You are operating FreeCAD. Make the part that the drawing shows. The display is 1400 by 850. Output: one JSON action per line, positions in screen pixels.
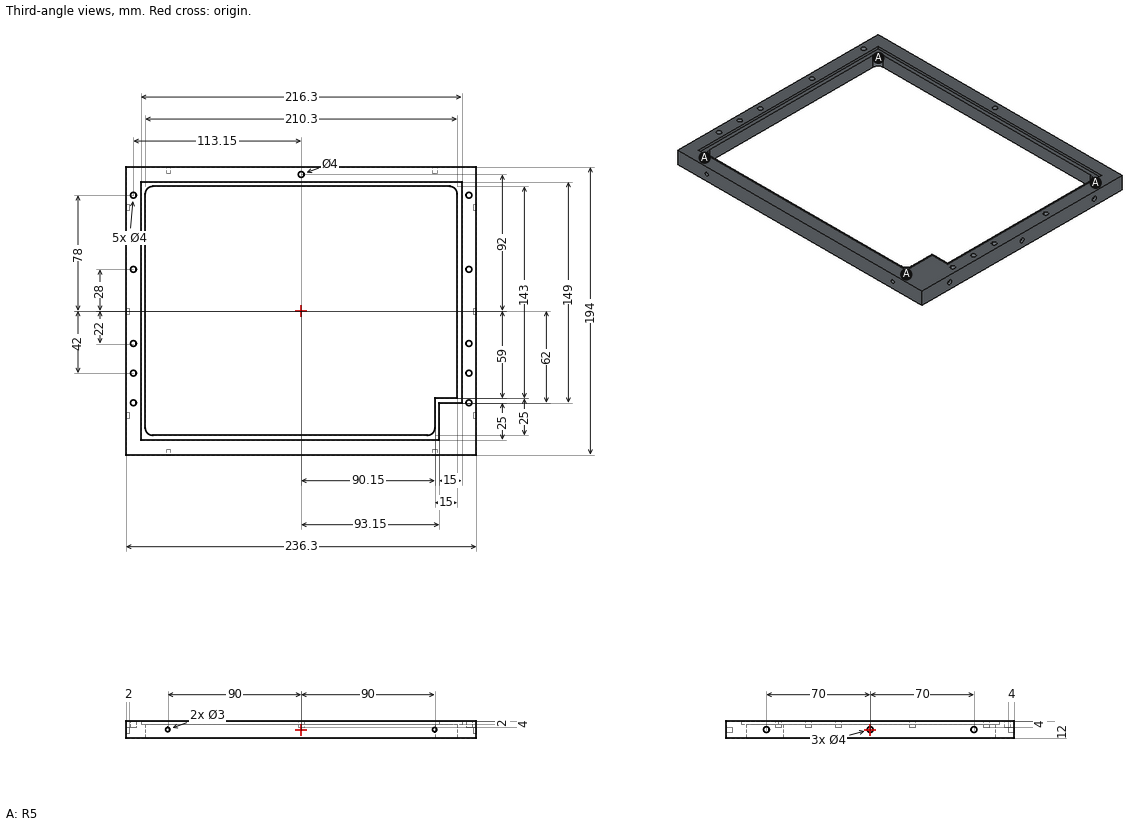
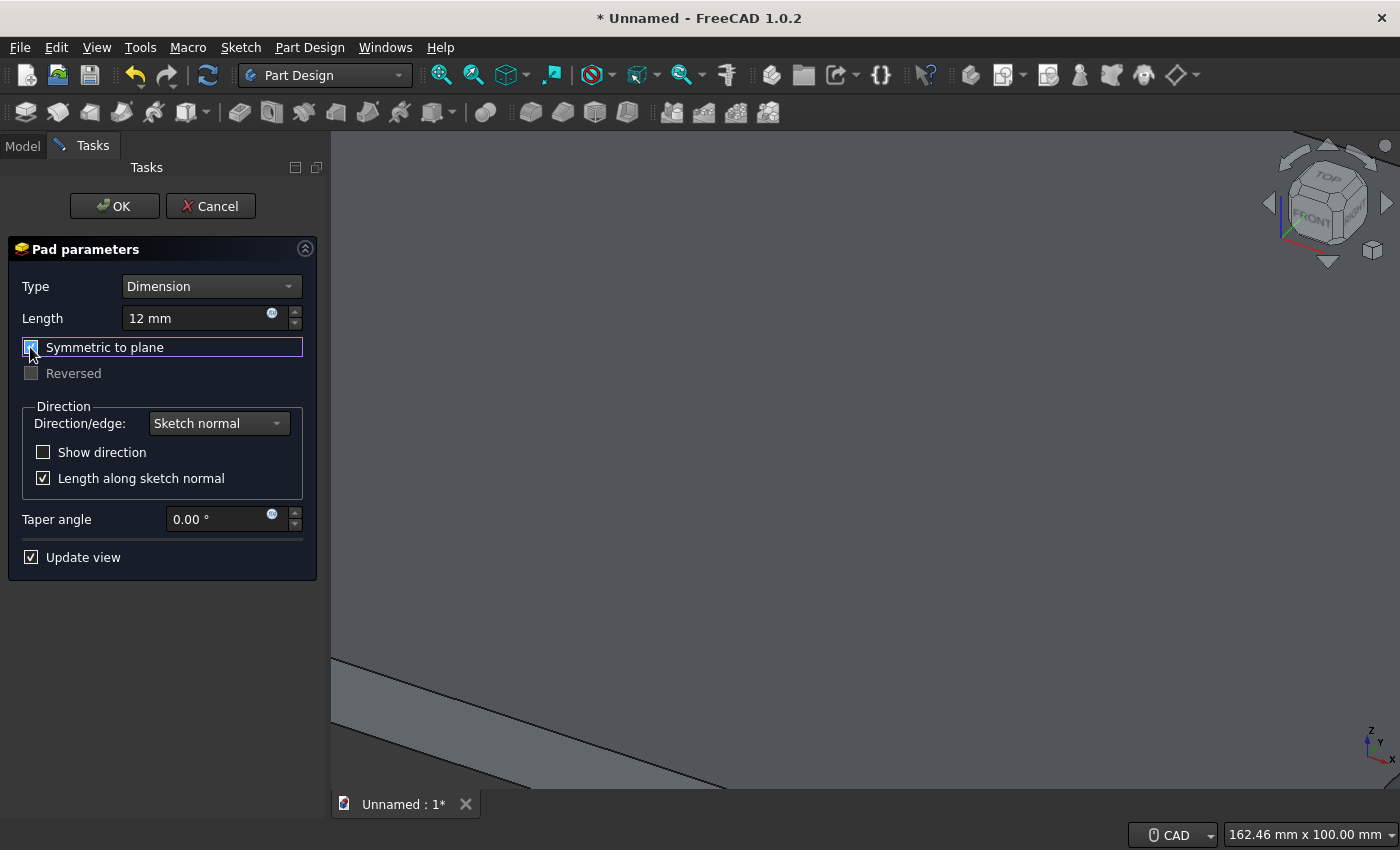
{"action": "left_click", "coordinate": [115, 206]}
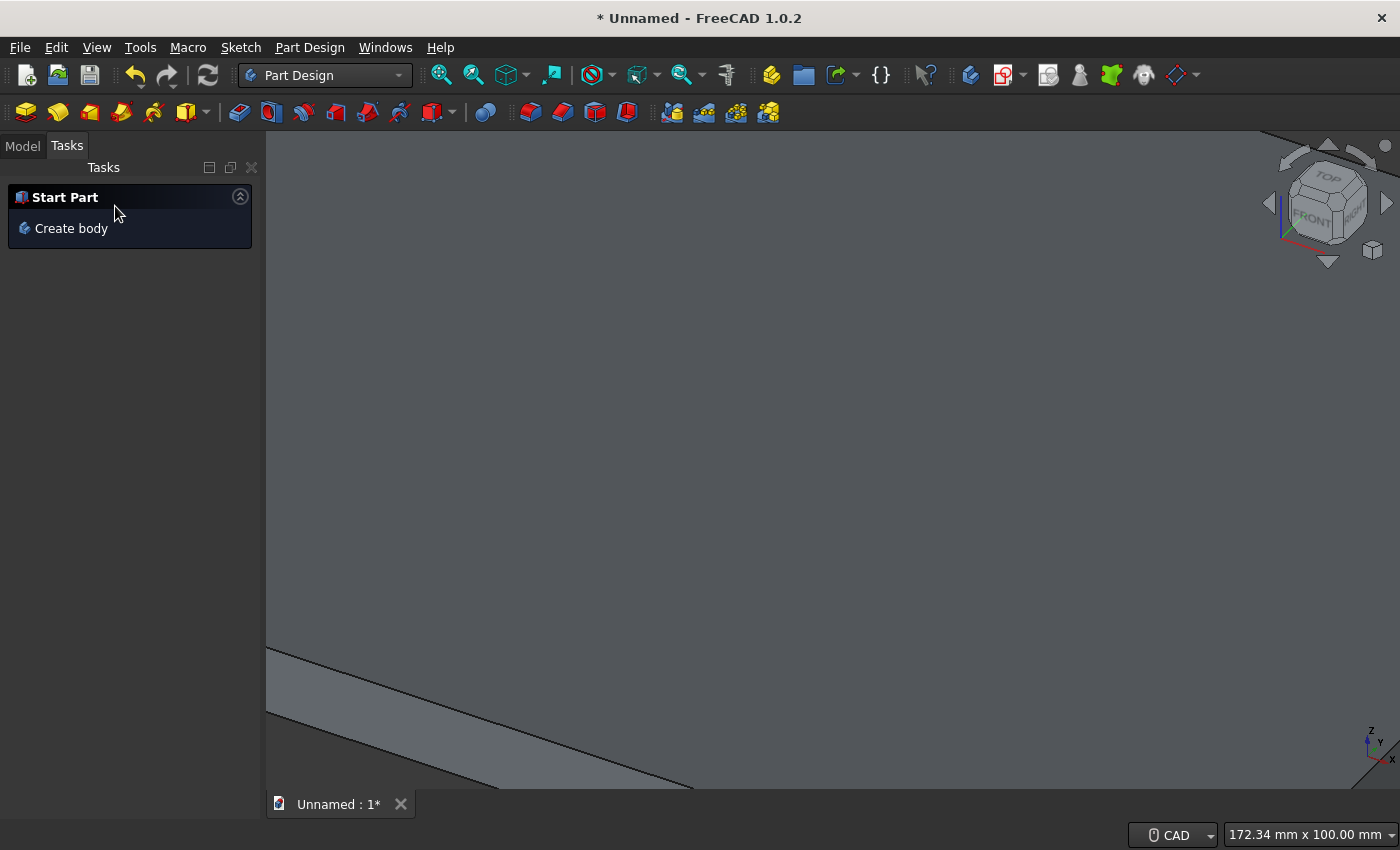
{"action": "left_click", "coordinate": [442, 76]}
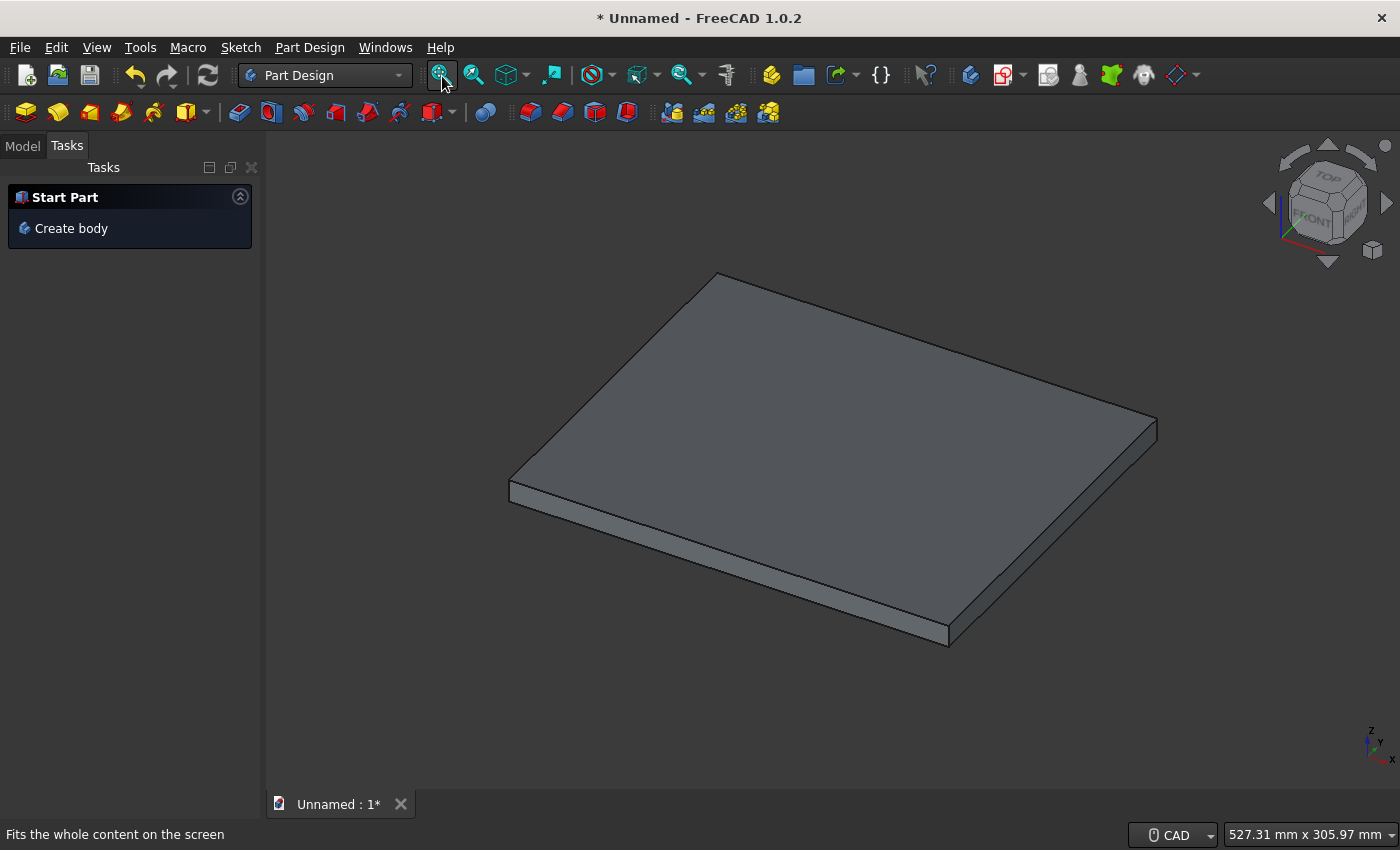
{"action": "left_click", "coordinate": [833, 448]}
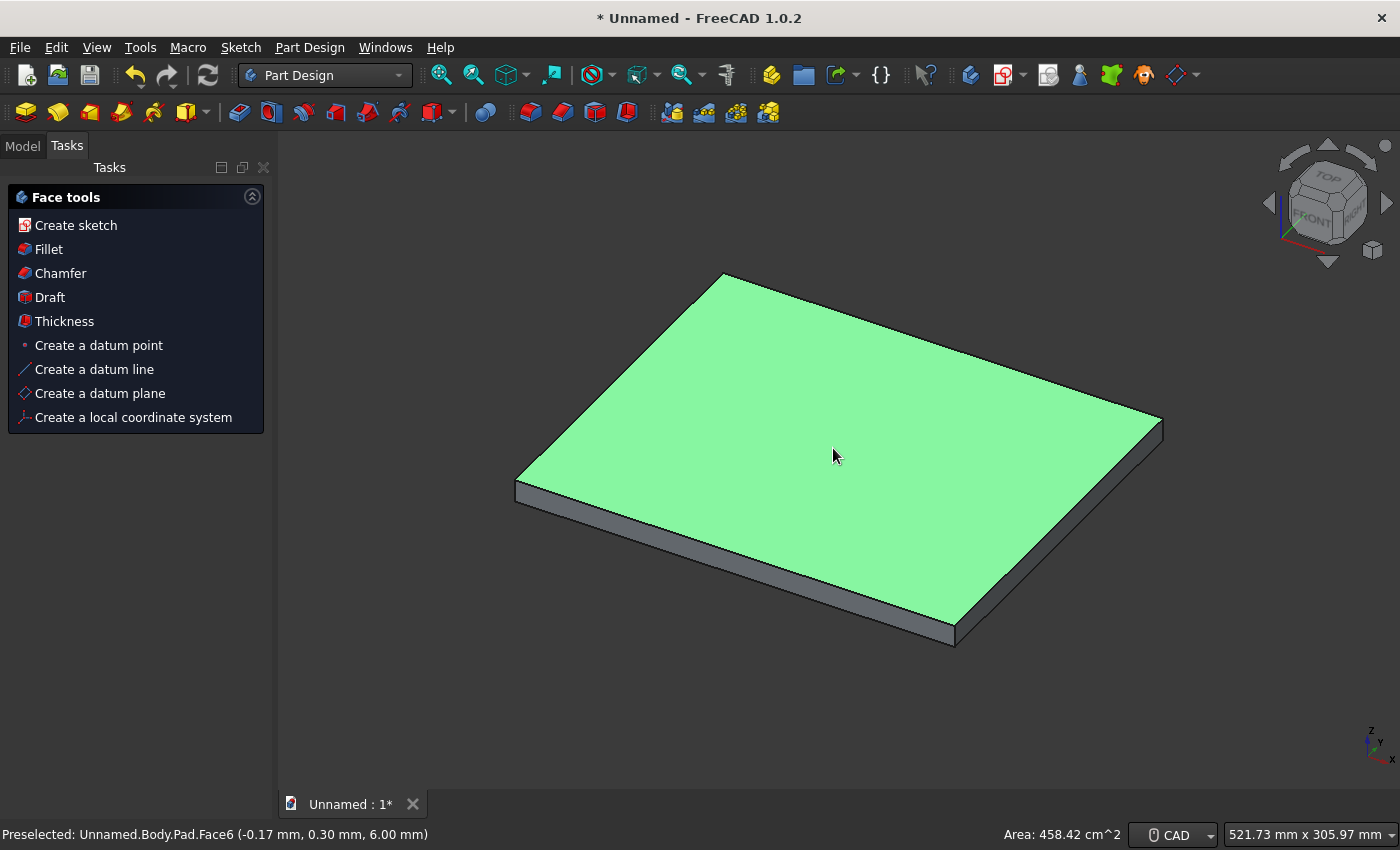
{"action": "left_click", "coordinate": [1004, 76]}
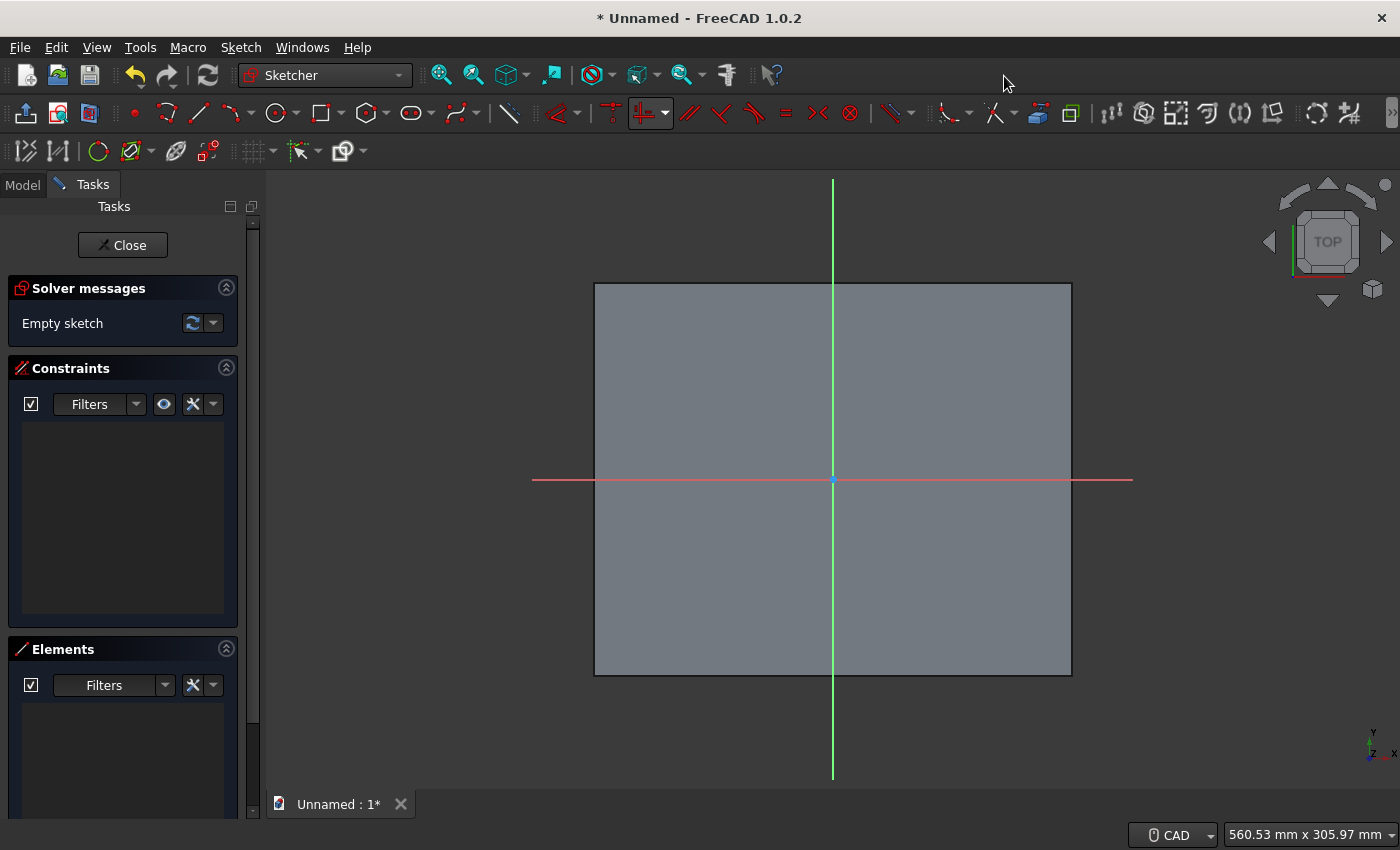
{"action": "left_click", "coordinate": [168, 114]}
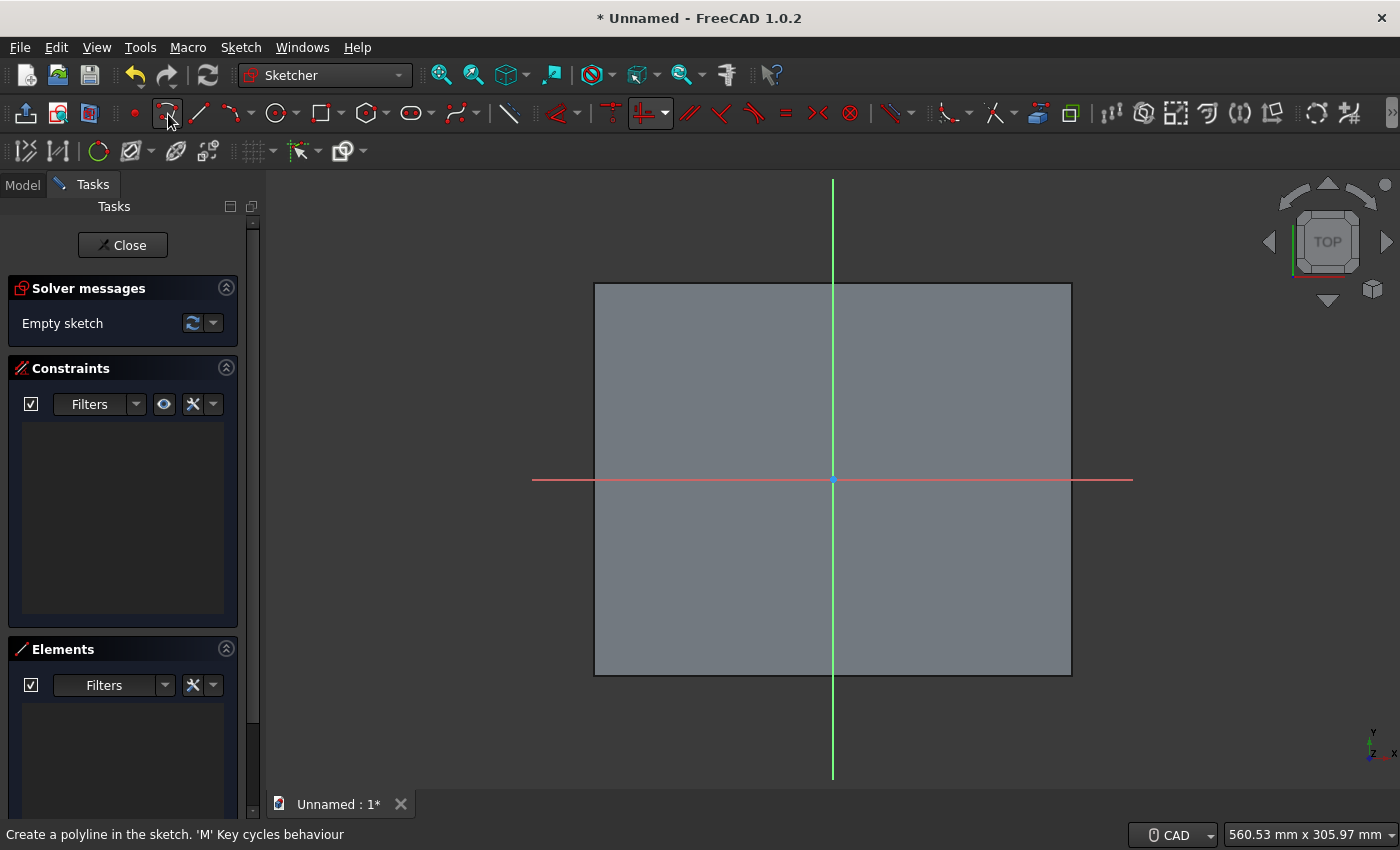
{"action": "left_click", "coordinate": [1021, 605]}
{"action": "left_click", "coordinate": [1052, 605]}
{"action": "left_click", "coordinate": [1052, 303]}
{"action": "left_click", "coordinate": [614, 303]}
{"action": "left_click", "coordinate": [614, 656]}
{"action": "left_click", "coordinate": [1021, 656]}
{"action": "left_click", "coordinate": [1021, 606]}
{"action": "key", "text": "Escape"}
{"action": "key", "text": "Escape"}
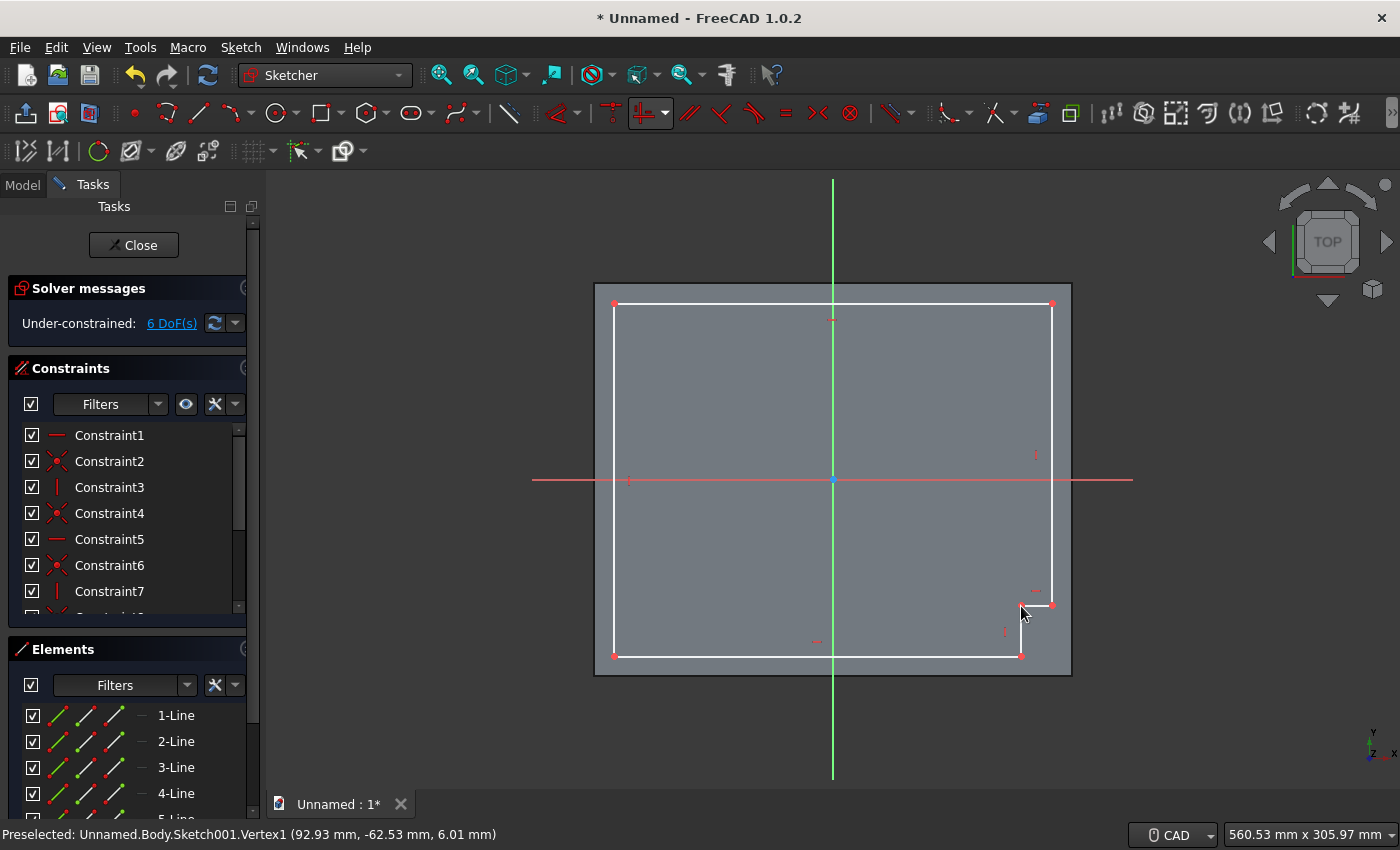
{"action": "left_click", "coordinate": [556, 114]}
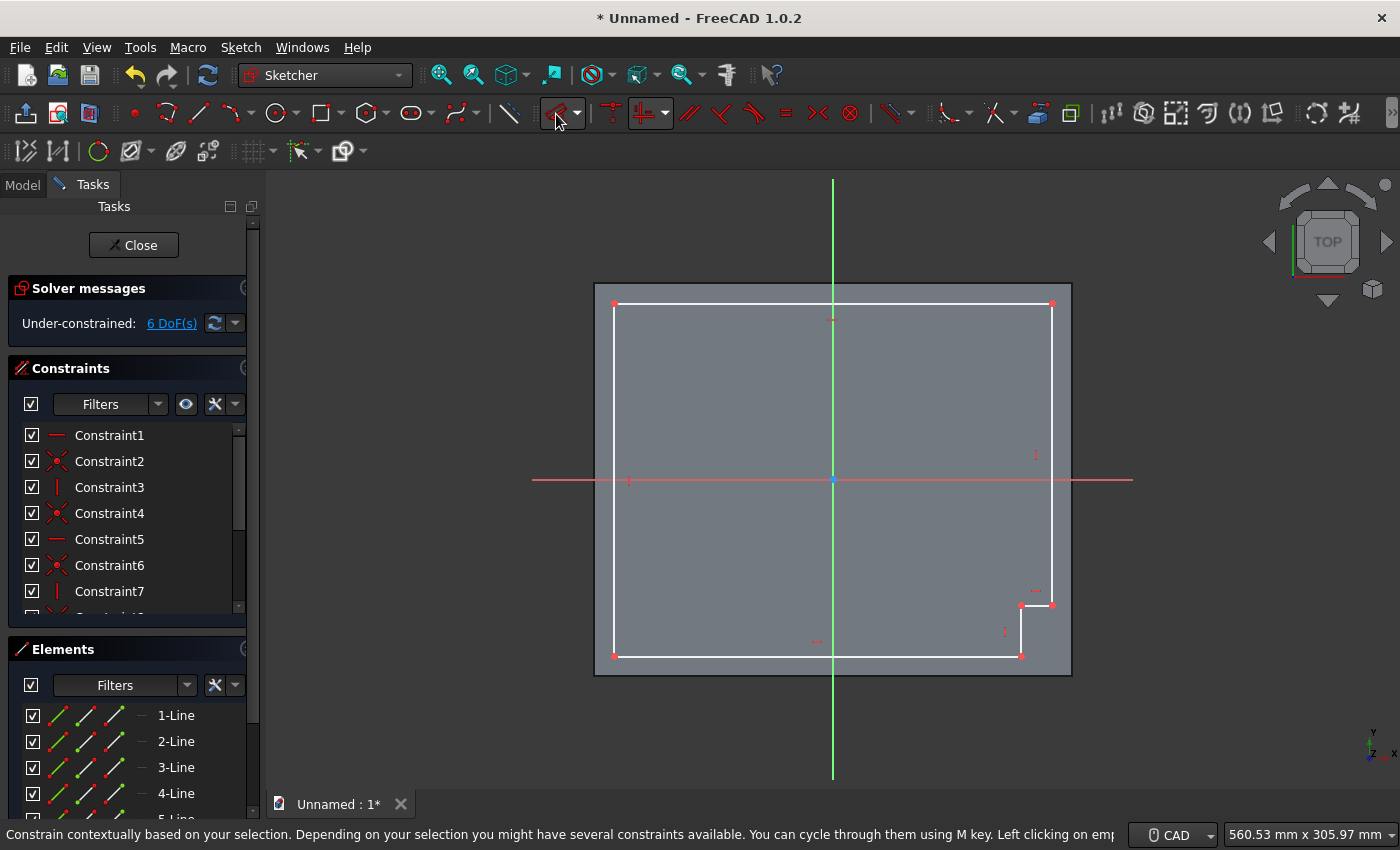
{"action": "scroll", "coordinate": [1030, 606], "scroll_direction": "up", "scroll_amount": 2}